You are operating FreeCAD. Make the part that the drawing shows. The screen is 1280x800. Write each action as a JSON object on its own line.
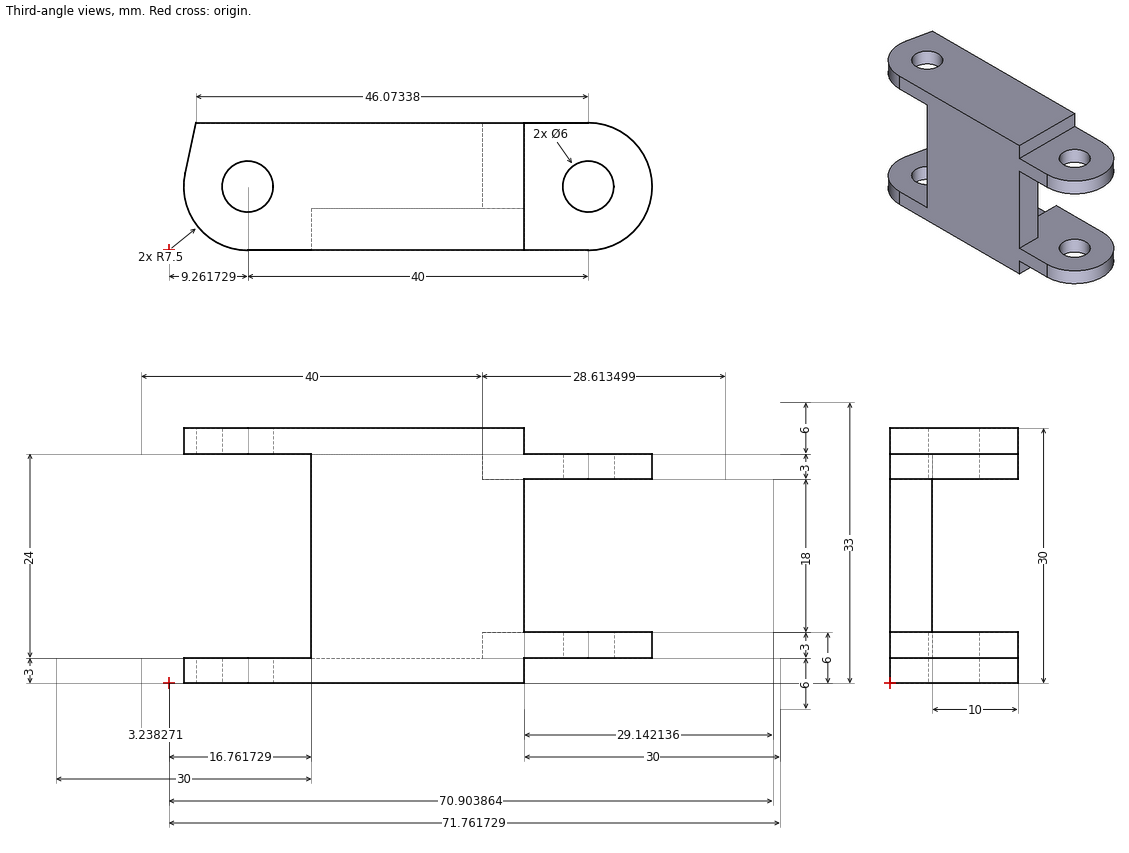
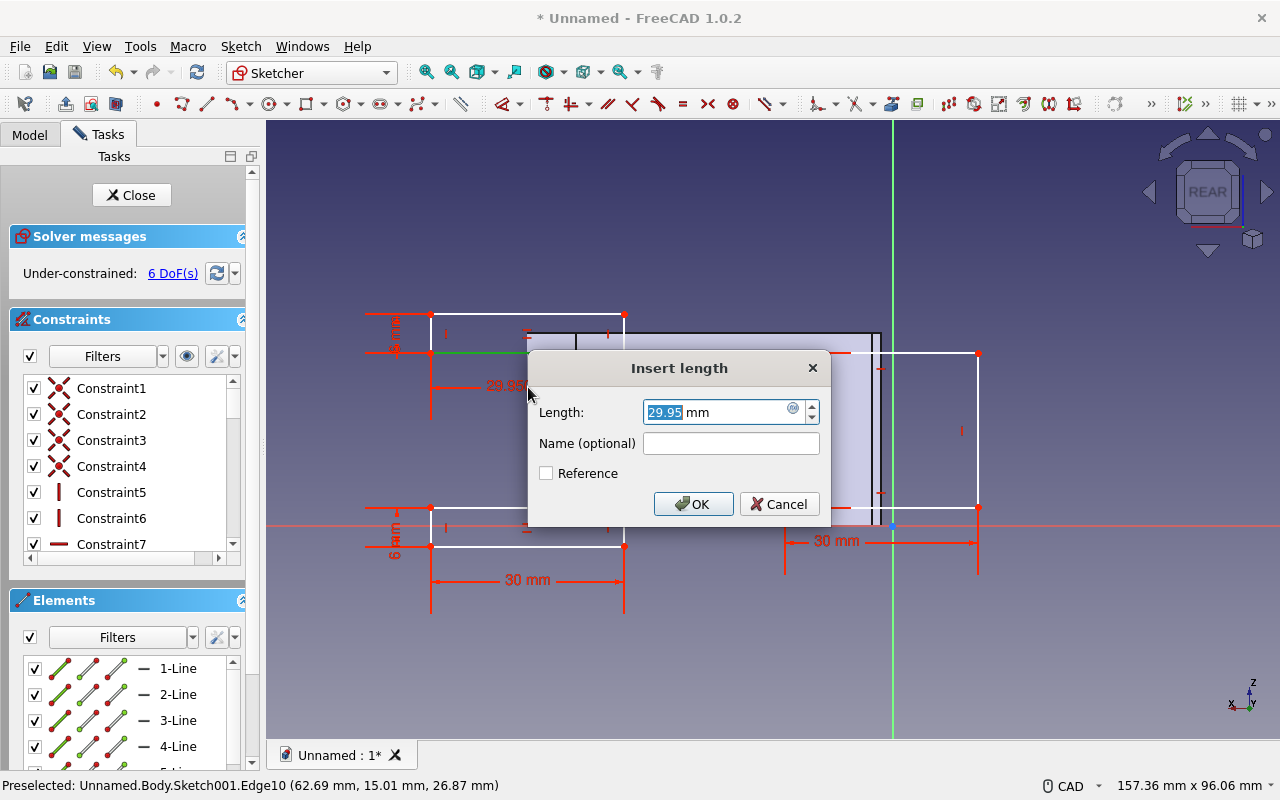
{"action": "type", "text": "30"}
{"action": "key", "text": "Return"}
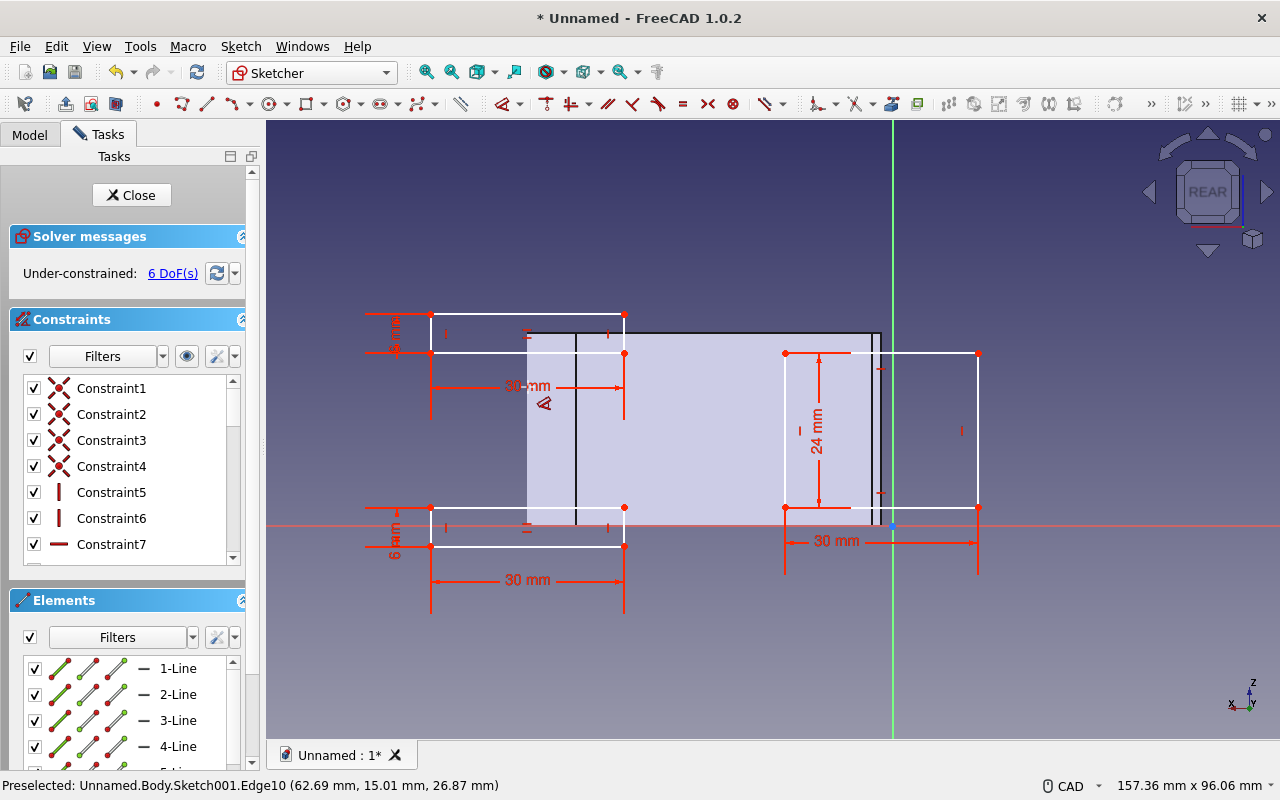
{"action": "scroll", "coordinate": [785, 508], "scroll_direction": "up", "scroll_amount": 4}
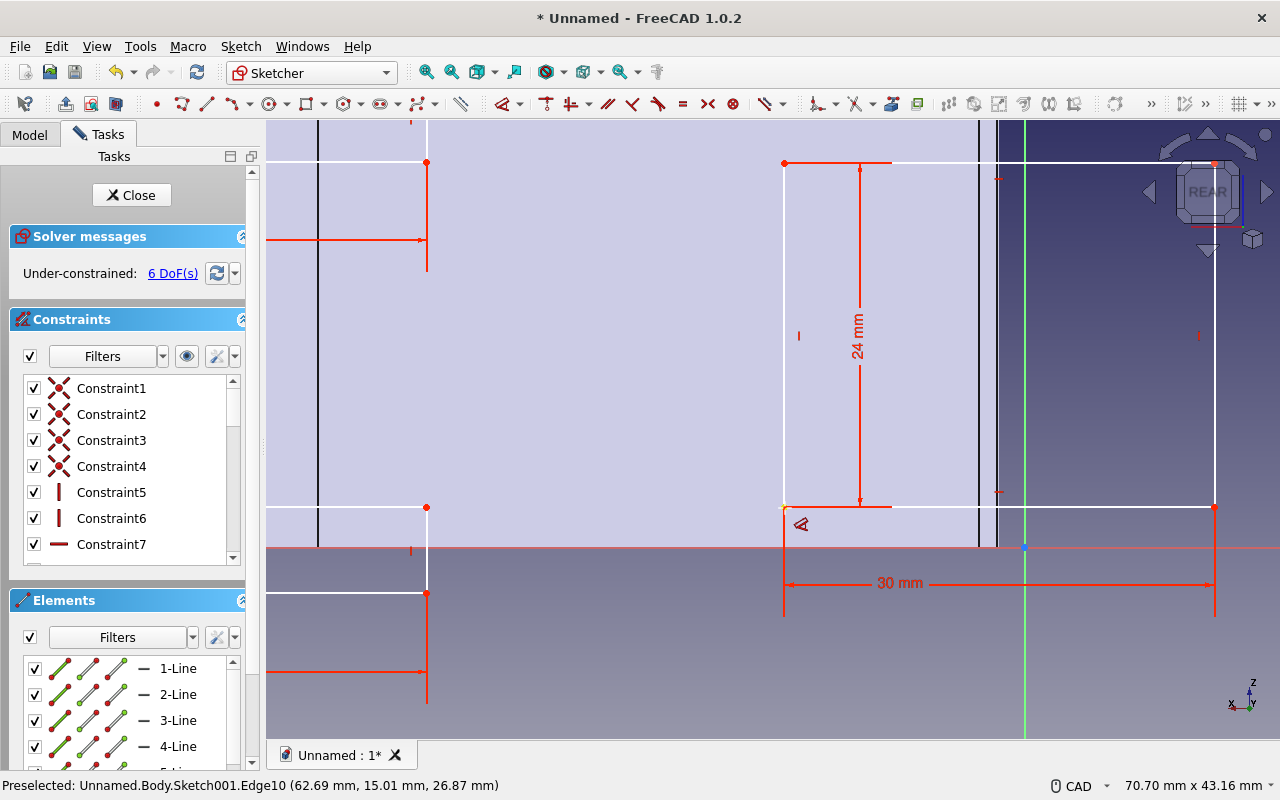
{"action": "left_click", "coordinate": [784, 507]}
{"action": "left_click", "coordinate": [1059, 527]}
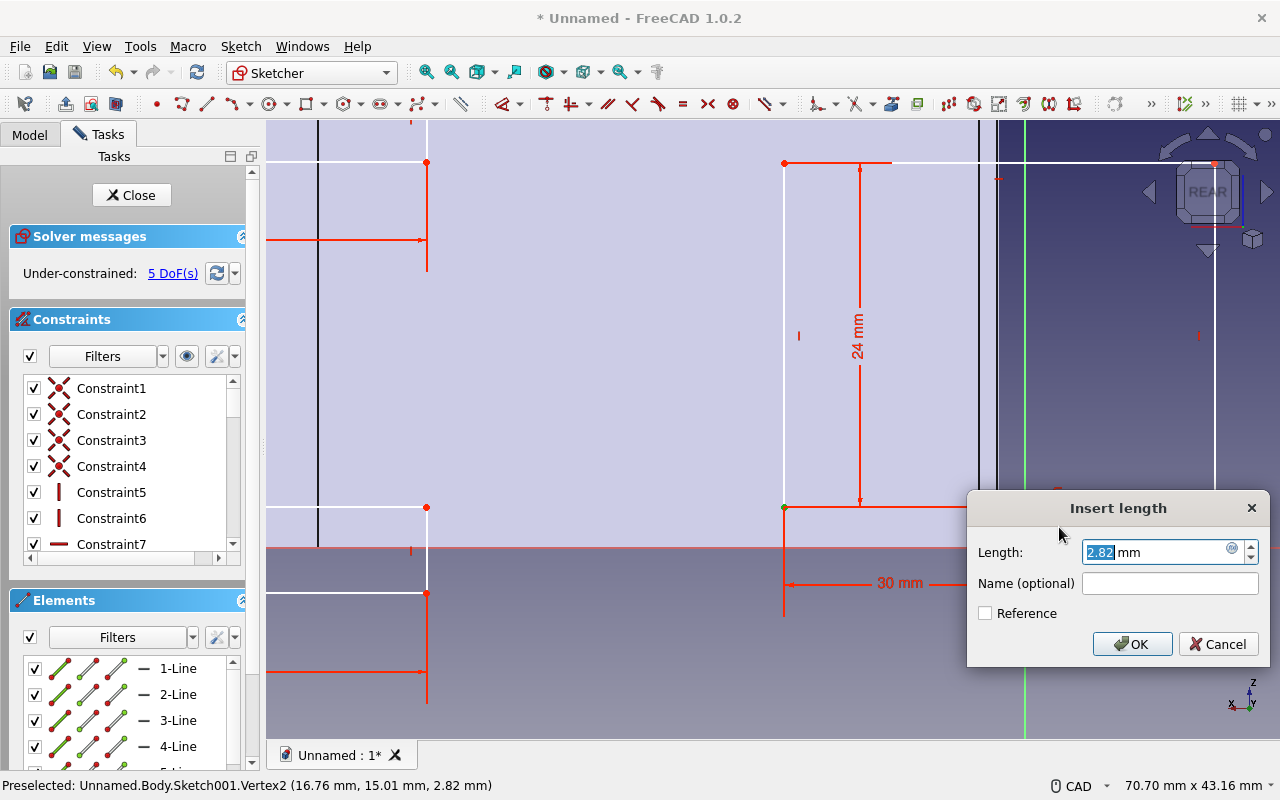
{"action": "type", "text": "3"}
{"action": "key", "text": "Return"}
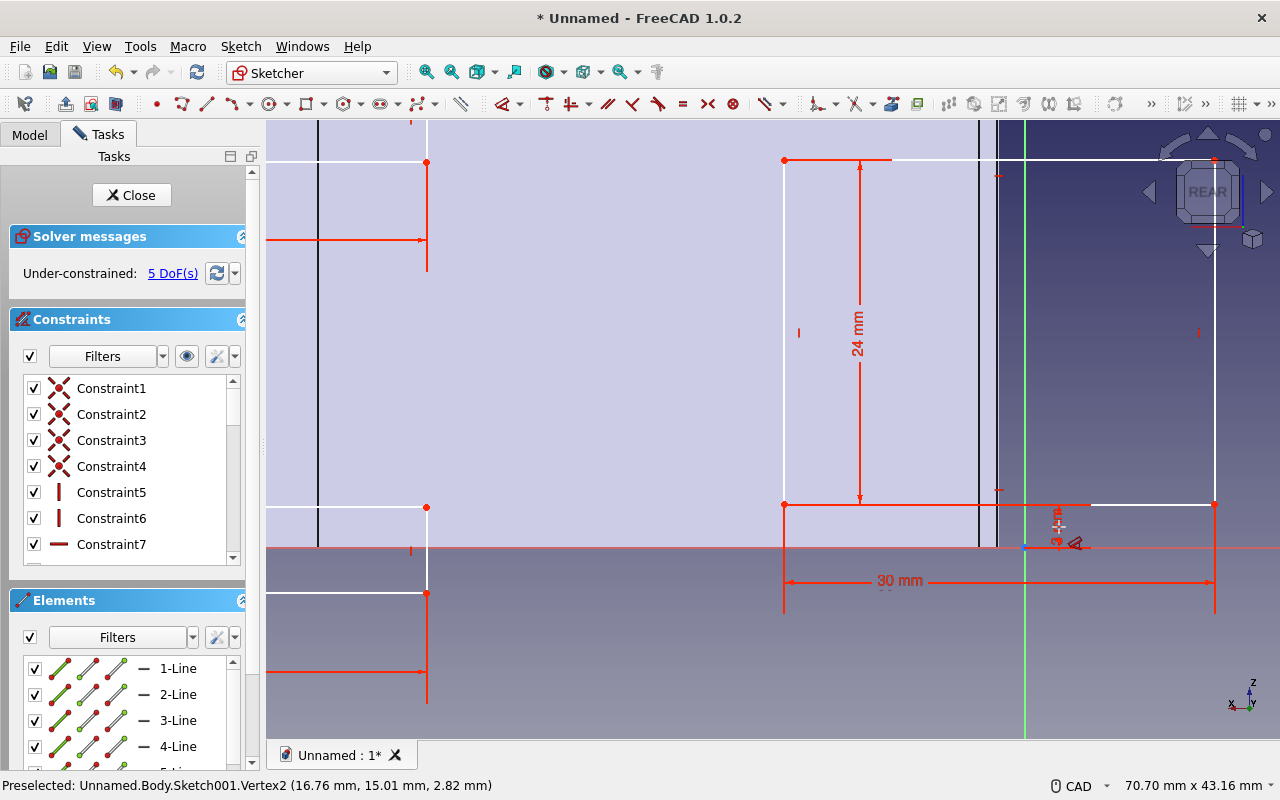
{"action": "scroll", "coordinate": [786, 509], "scroll_direction": "down", "scroll_amount": 4}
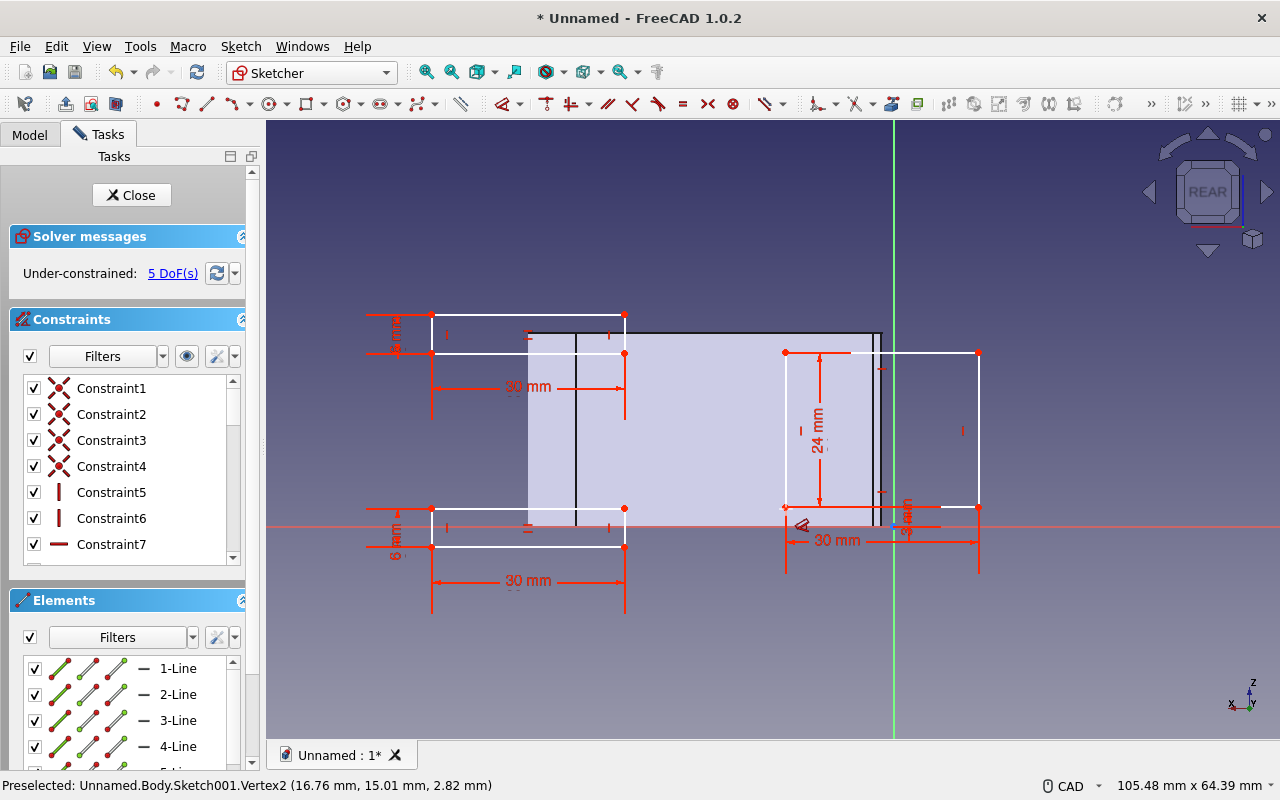
{"action": "scroll", "coordinate": [432, 509], "scroll_direction": "up", "scroll_amount": 4}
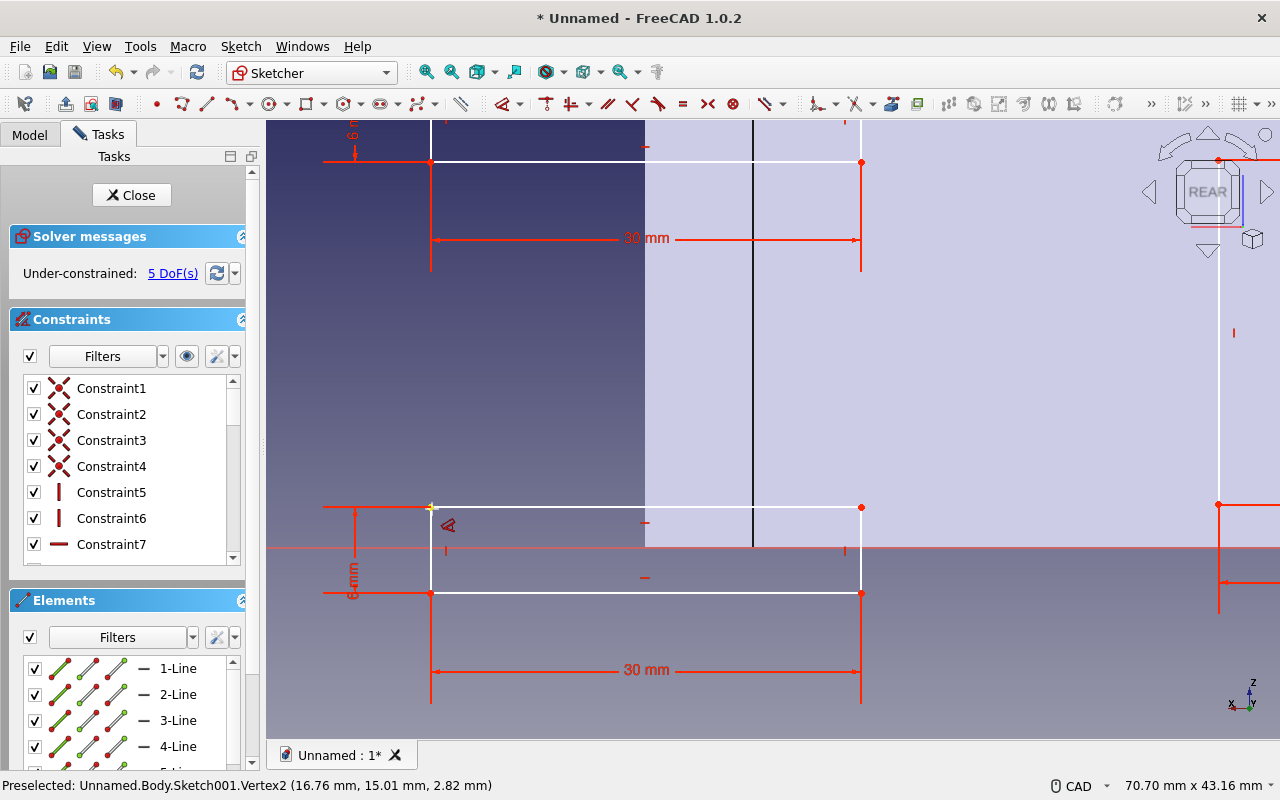
{"action": "left_click", "coordinate": [431, 507]}
{"action": "left_click", "coordinate": [397, 527]}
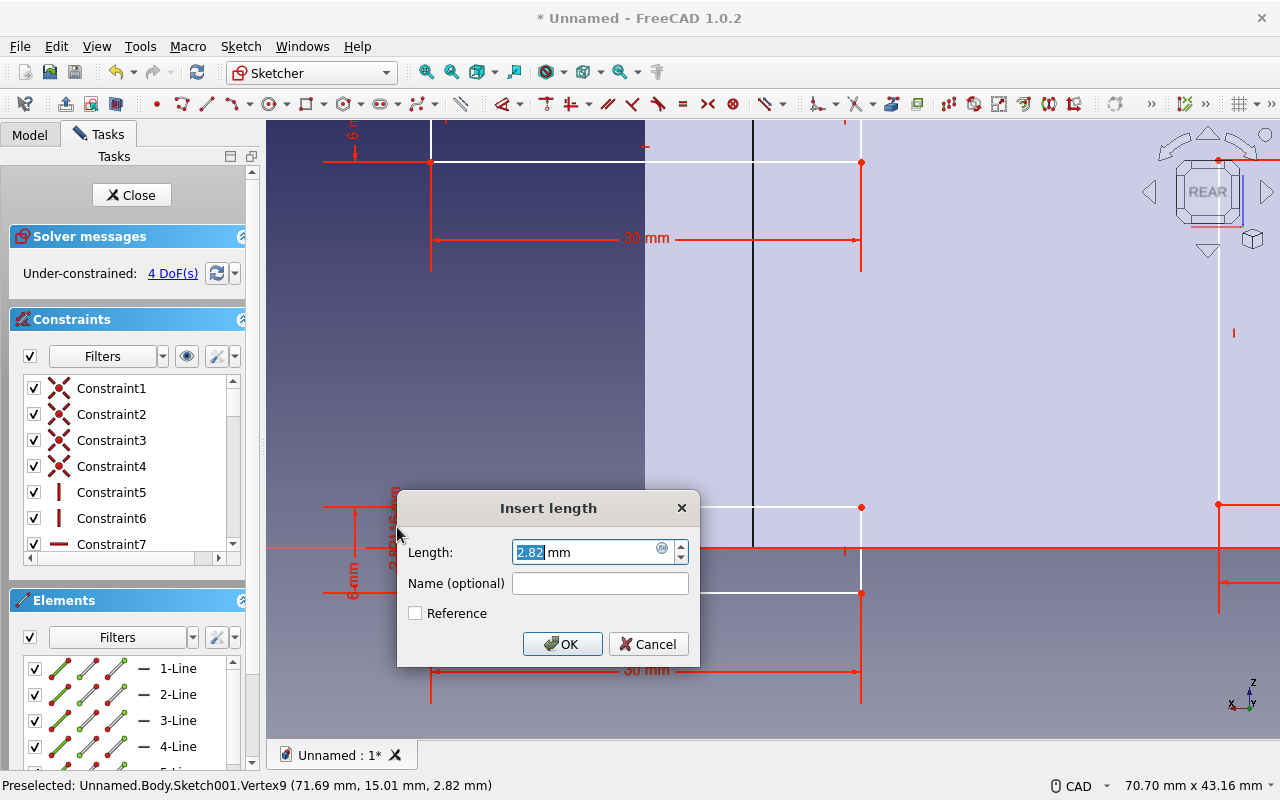
{"action": "type", "text": "3"}
{"action": "key", "text": "Return"}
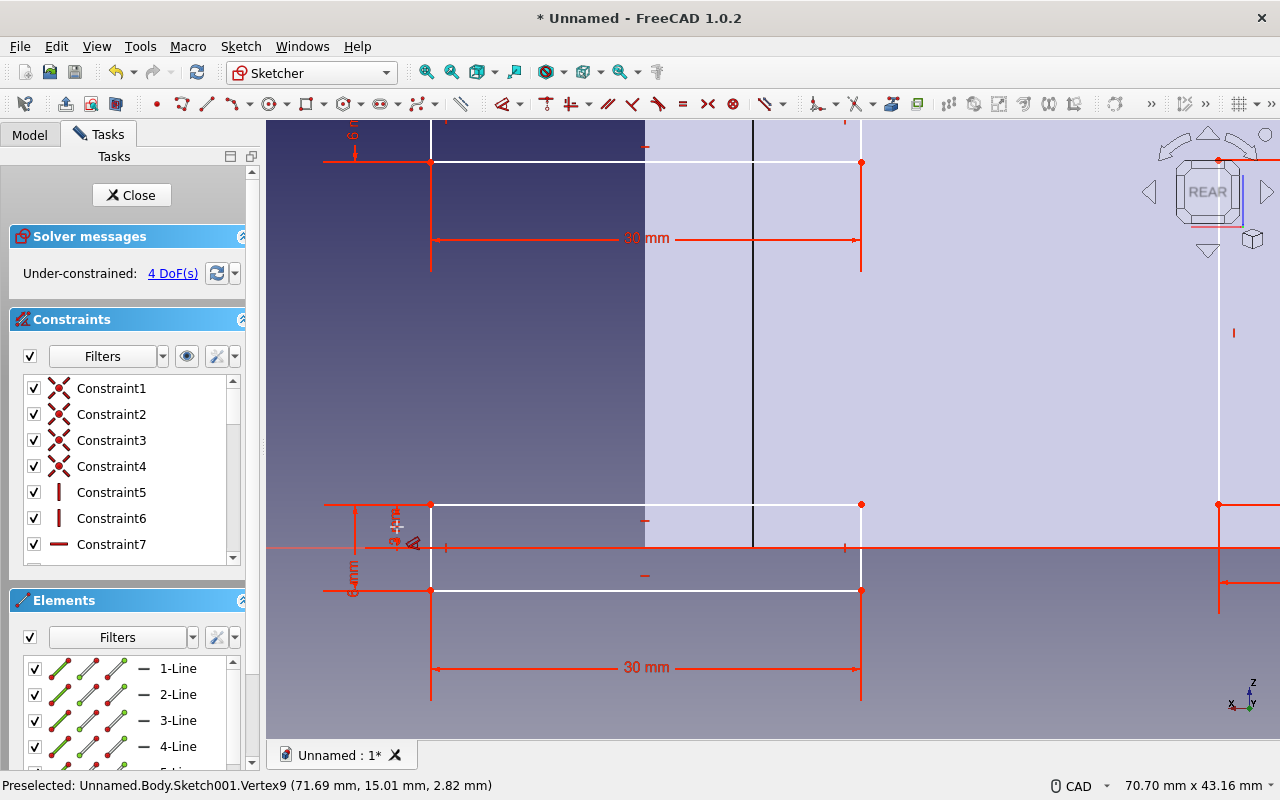
{"action": "scroll", "coordinate": [431, 509], "scroll_direction": "down", "scroll_amount": 4}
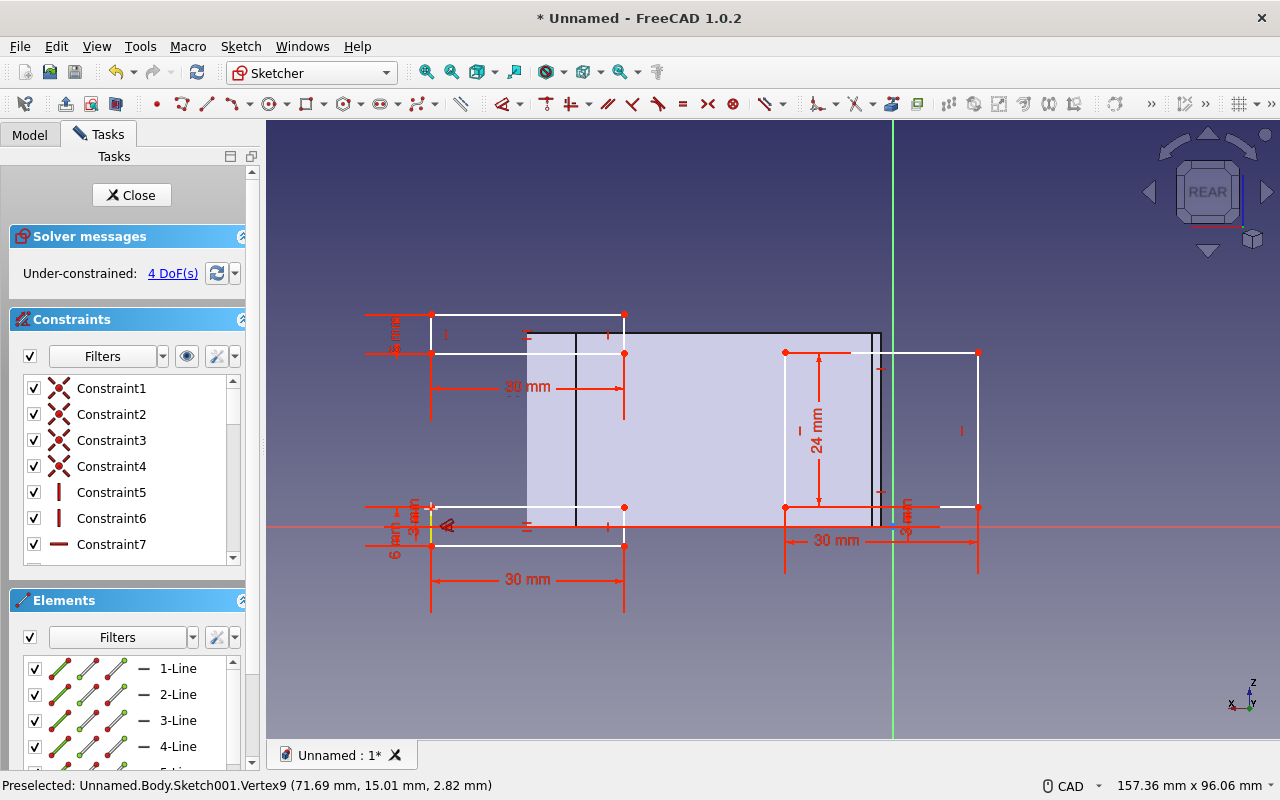
{"action": "left_click", "coordinate": [431, 315]}
{"action": "left_click", "coordinate": [397, 421]}